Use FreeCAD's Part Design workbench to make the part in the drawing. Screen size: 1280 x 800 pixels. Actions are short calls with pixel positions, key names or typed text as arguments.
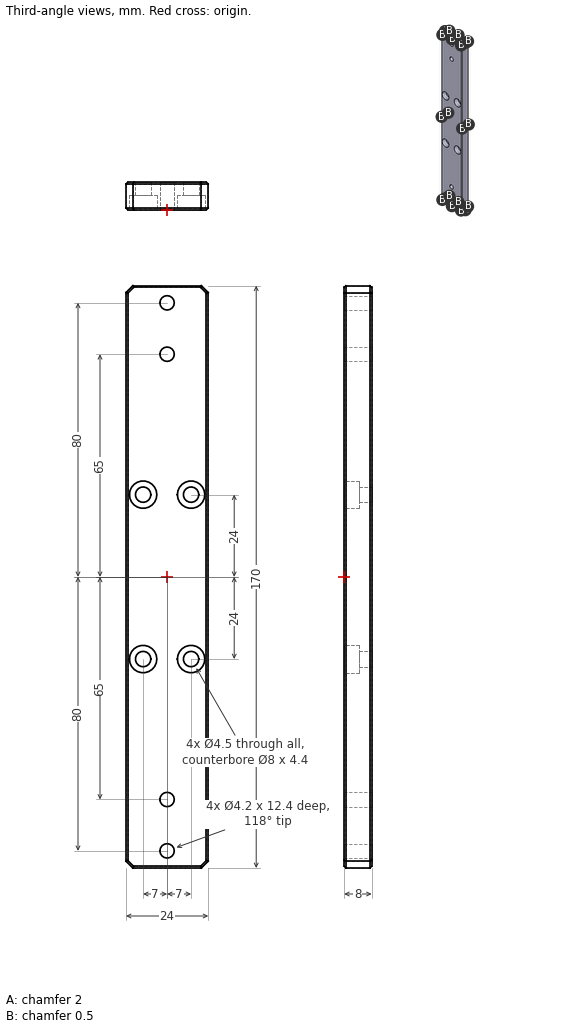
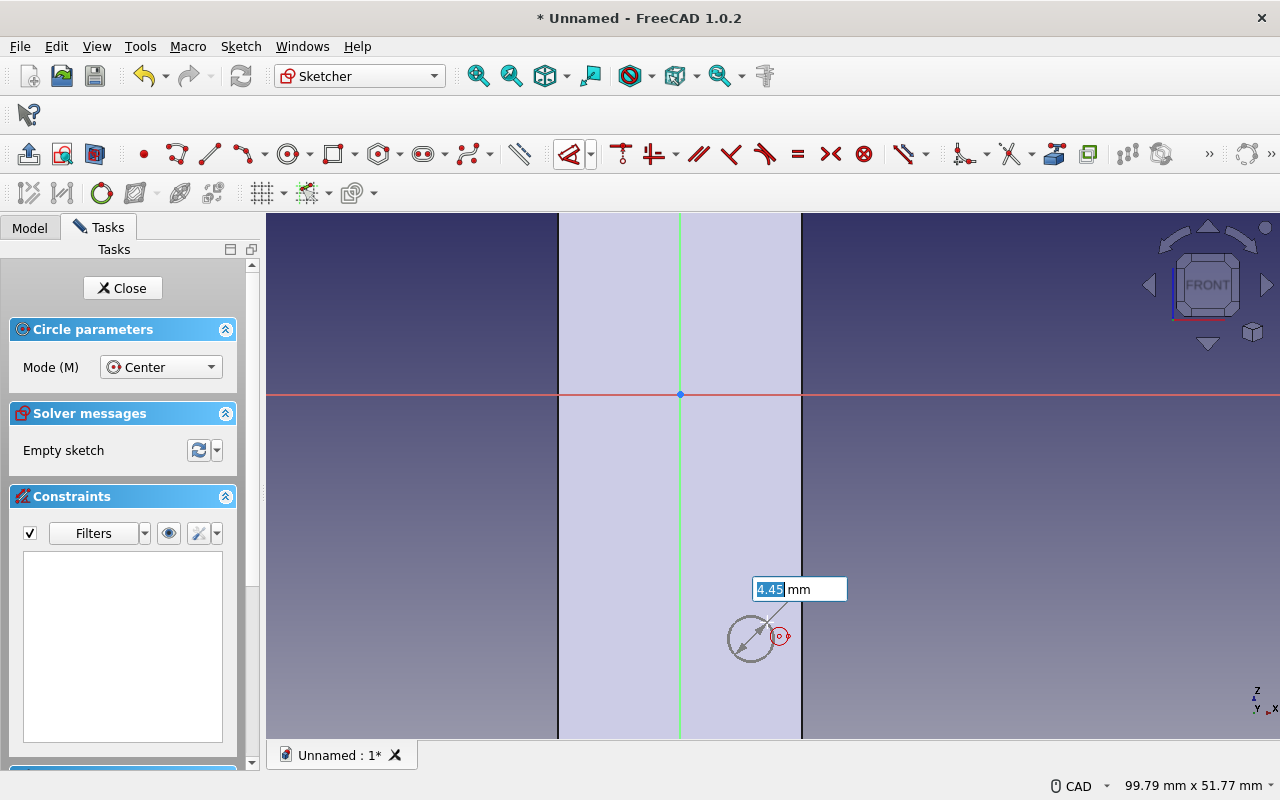
text(4.5)
key(Return)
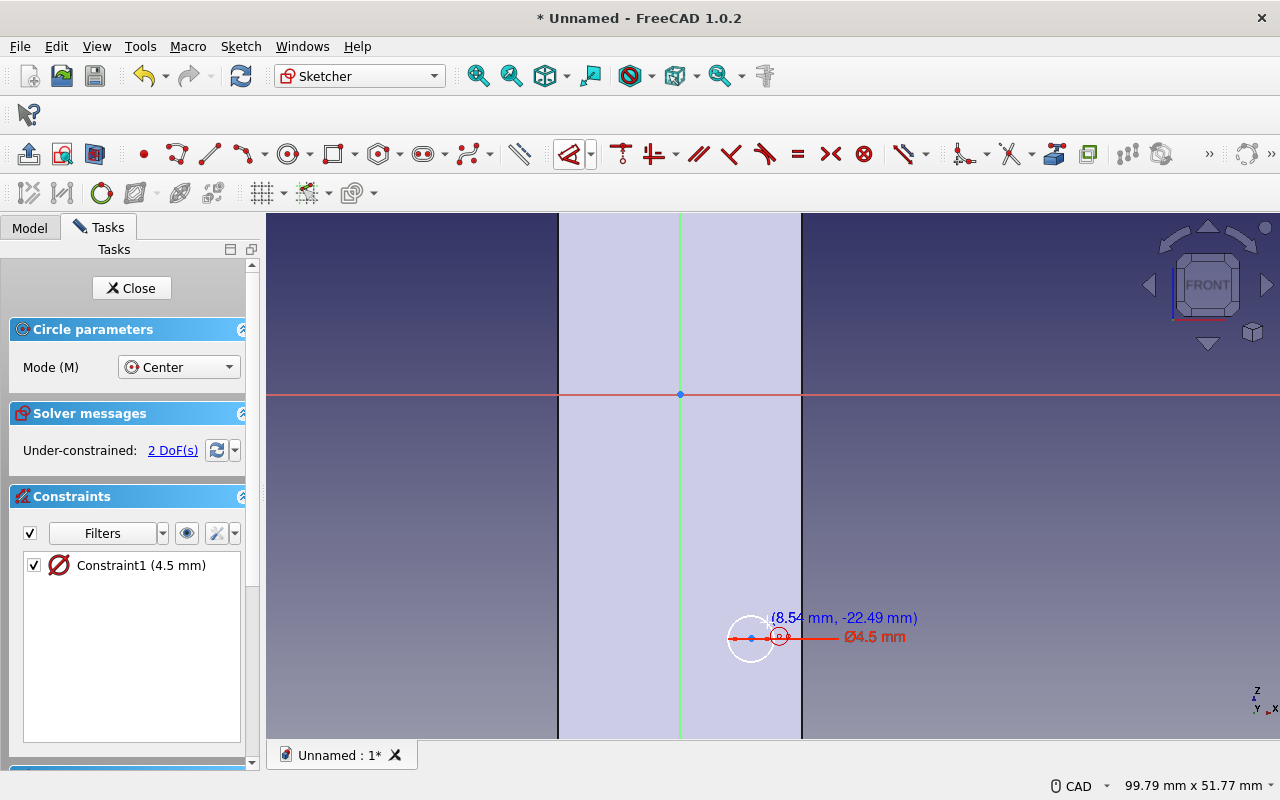
click(609, 638)
move(625, 622)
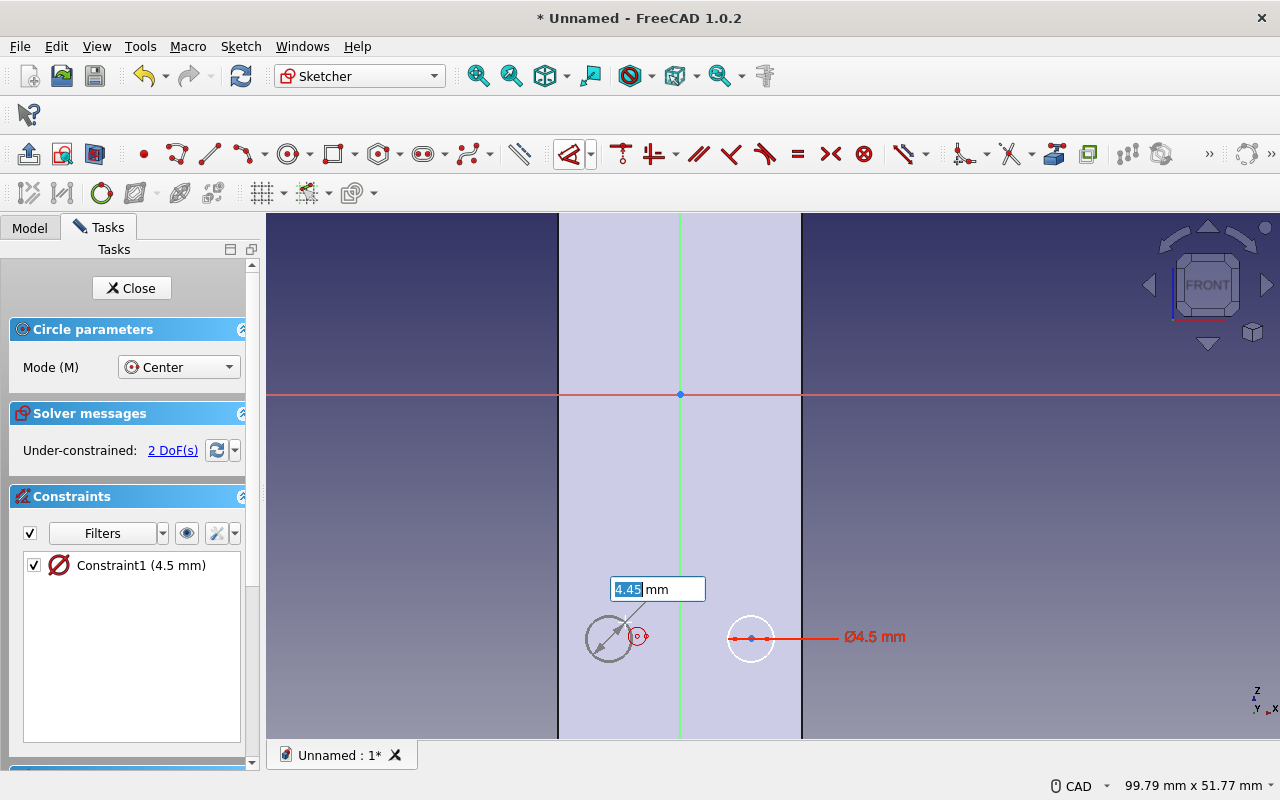
text(4.5)
key(Return)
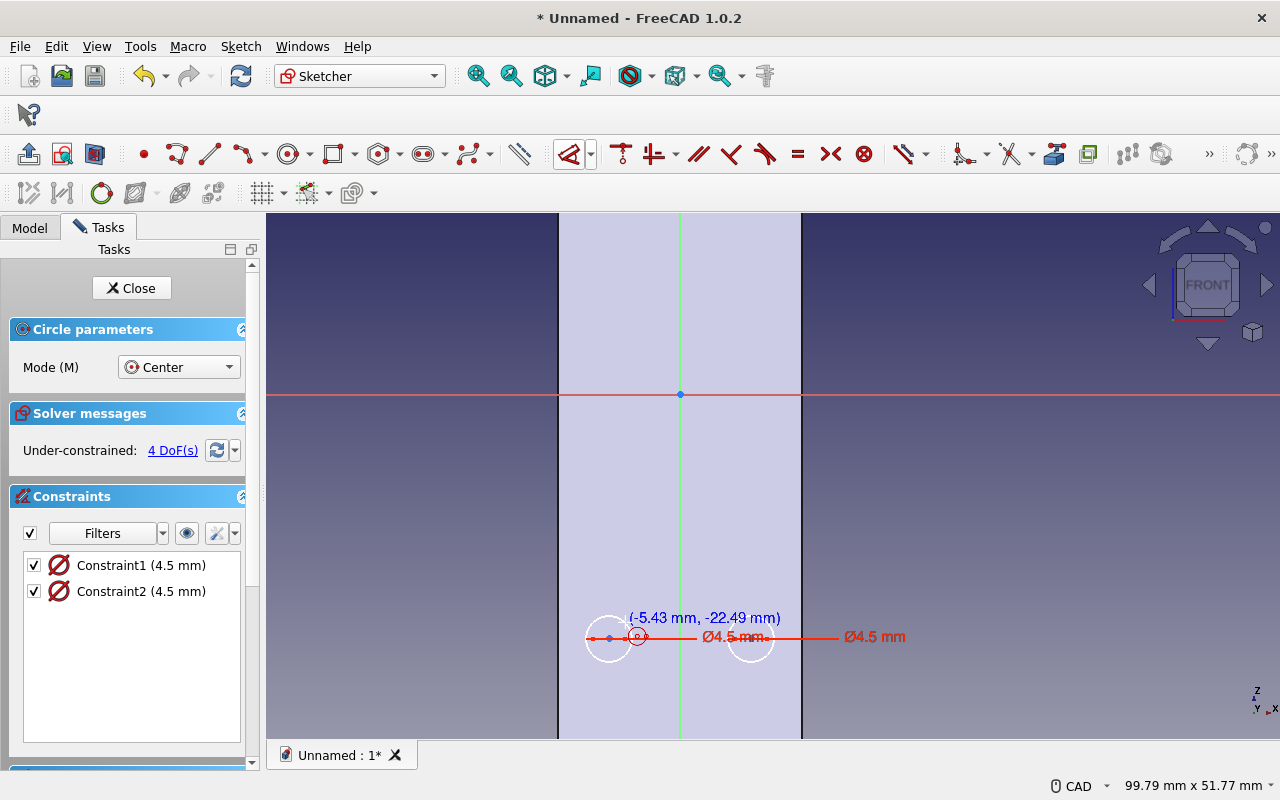
scroll(754, 642, down, 2)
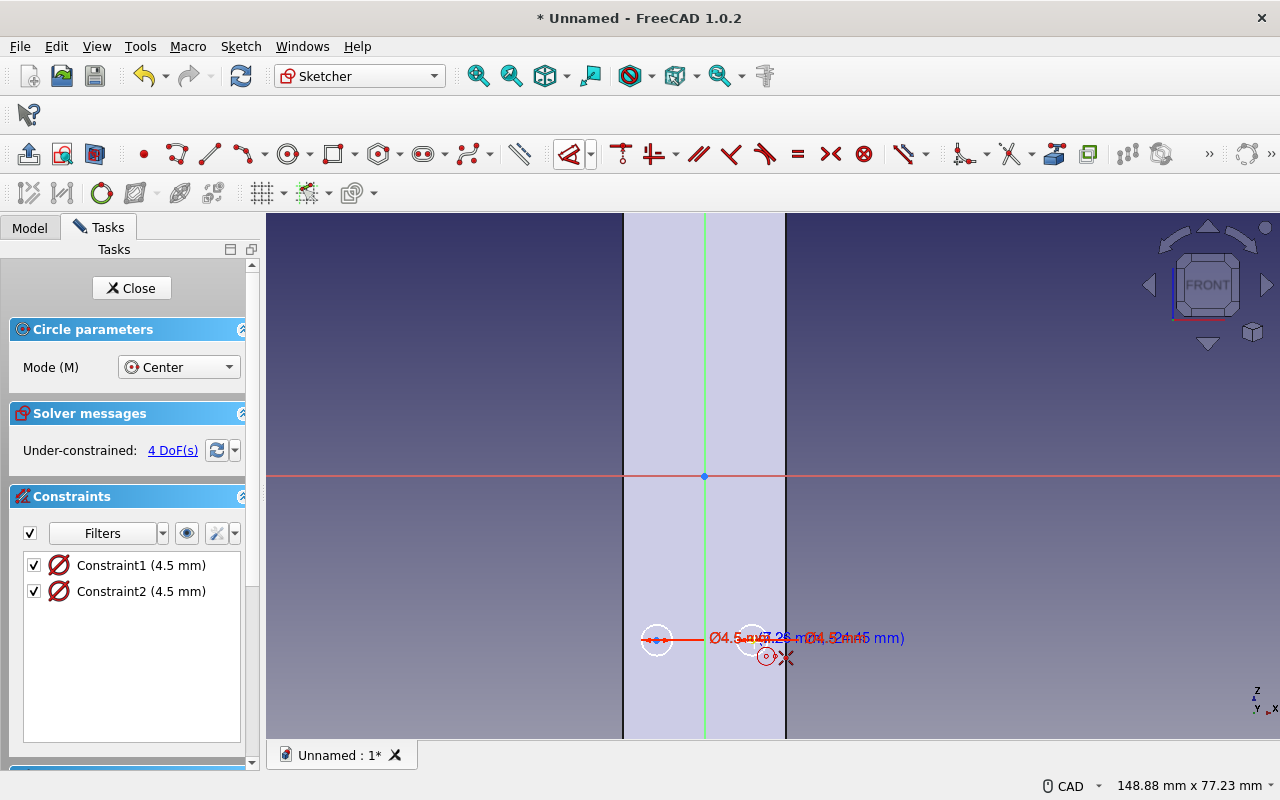
scroll(752, 313, up, 2)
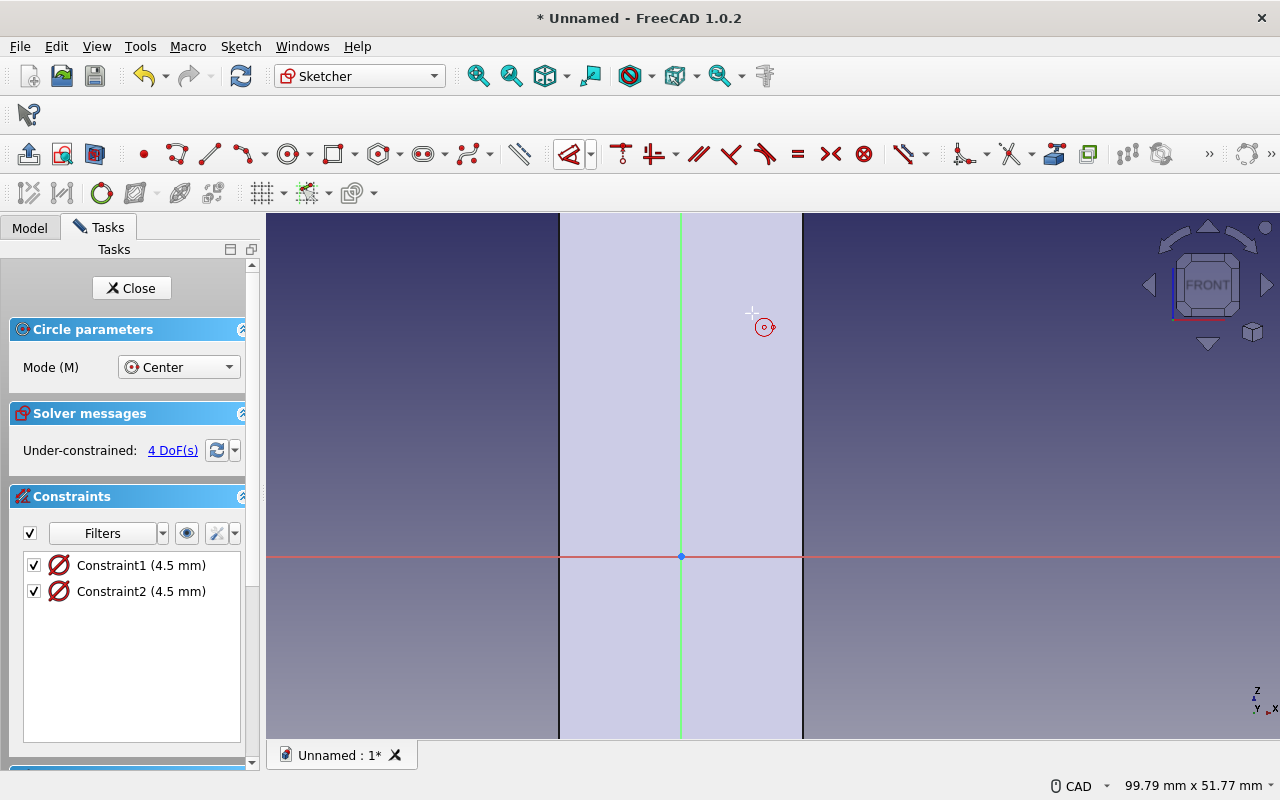
click(752, 313)
move(768, 297)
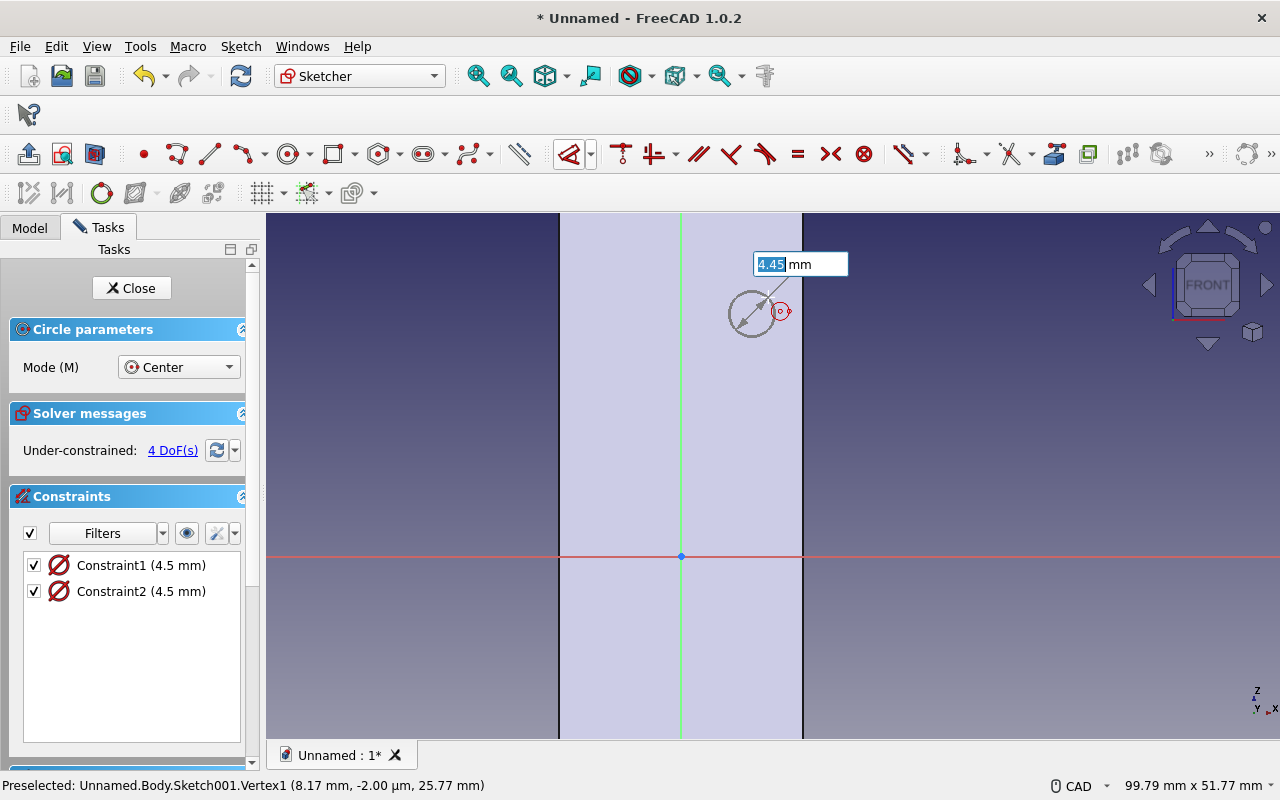
text(4.5)
key(Return)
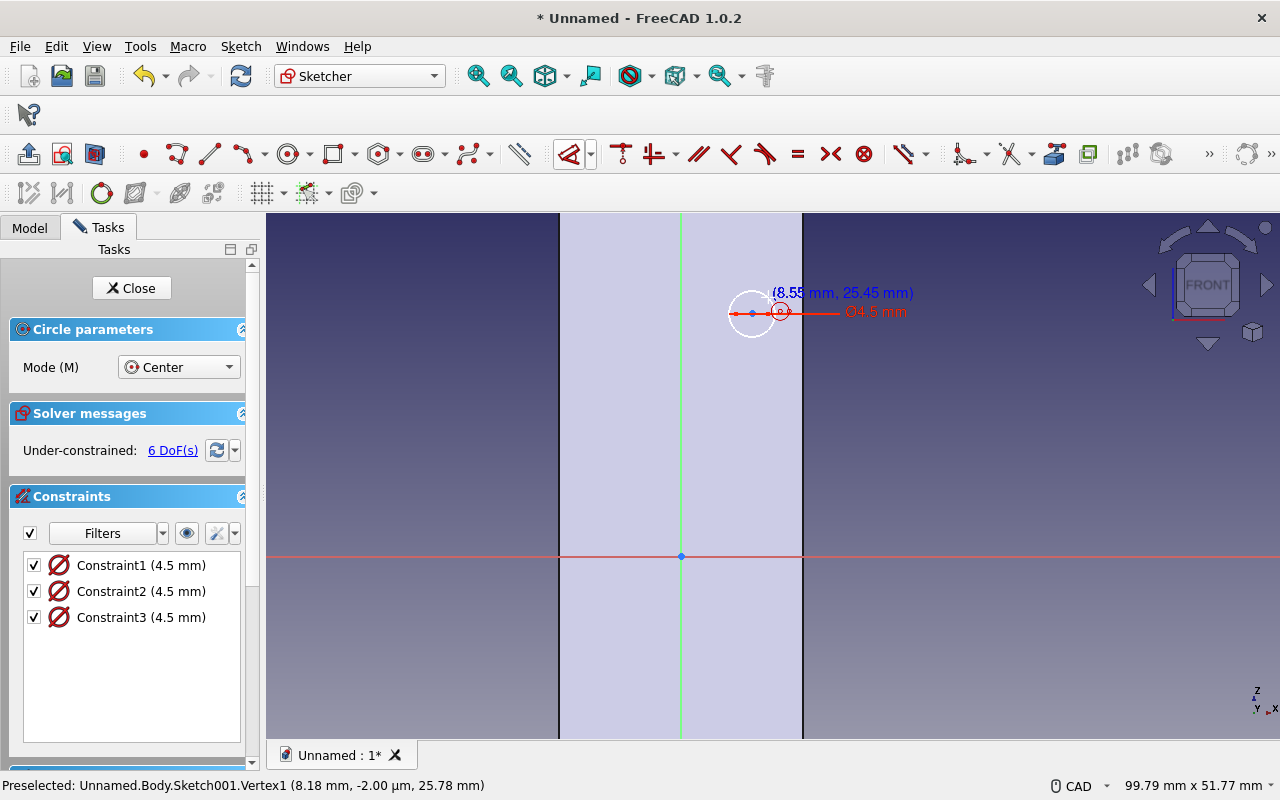
click(610, 313)
move(626, 297)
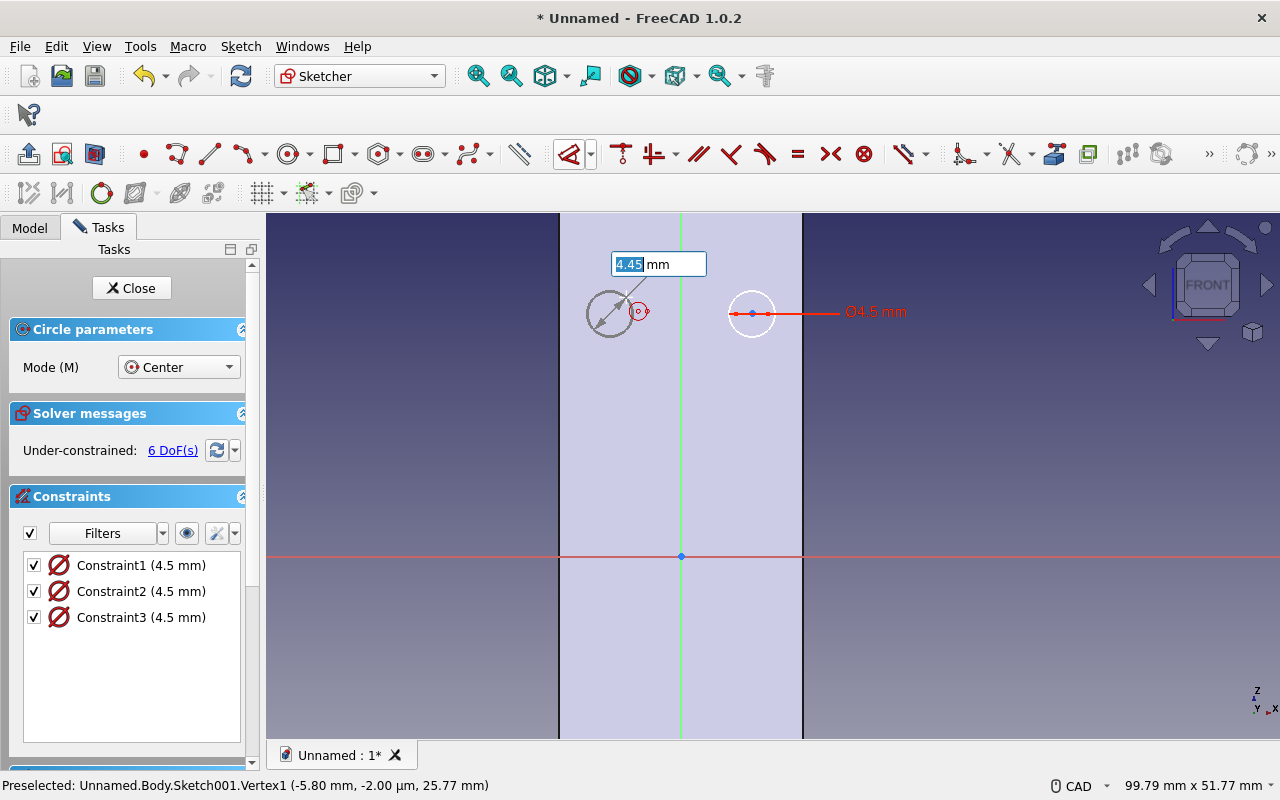
text(4.5)
key(Return)
key(Escape)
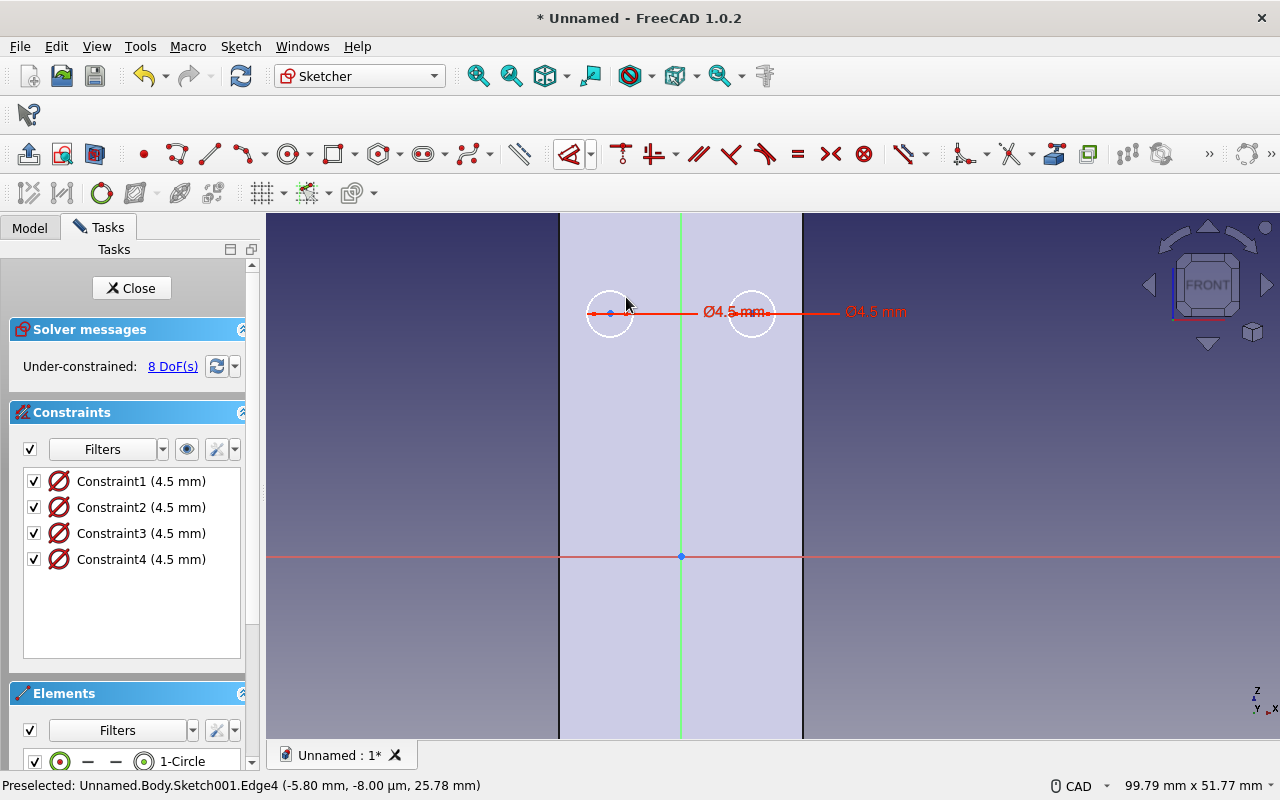
scroll(752, 312, down, 2)